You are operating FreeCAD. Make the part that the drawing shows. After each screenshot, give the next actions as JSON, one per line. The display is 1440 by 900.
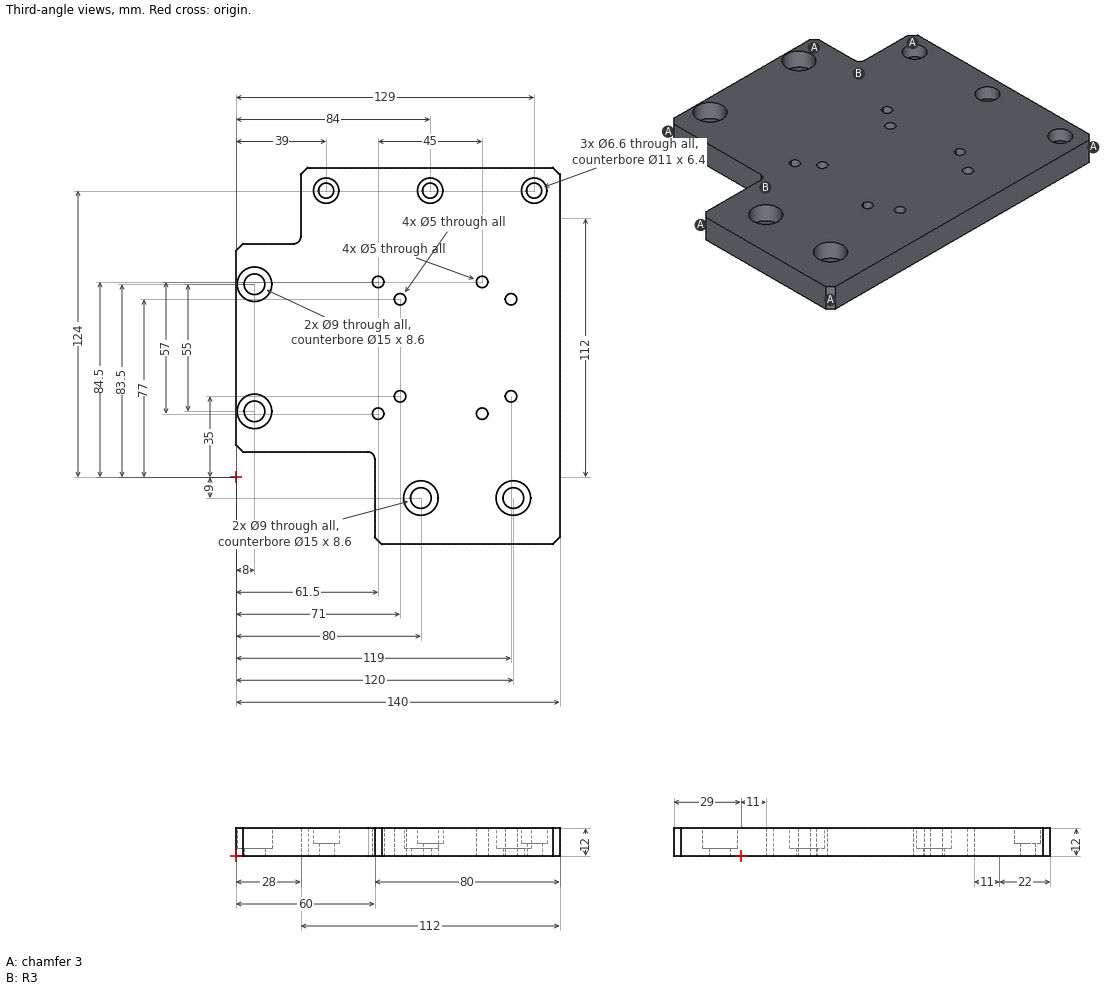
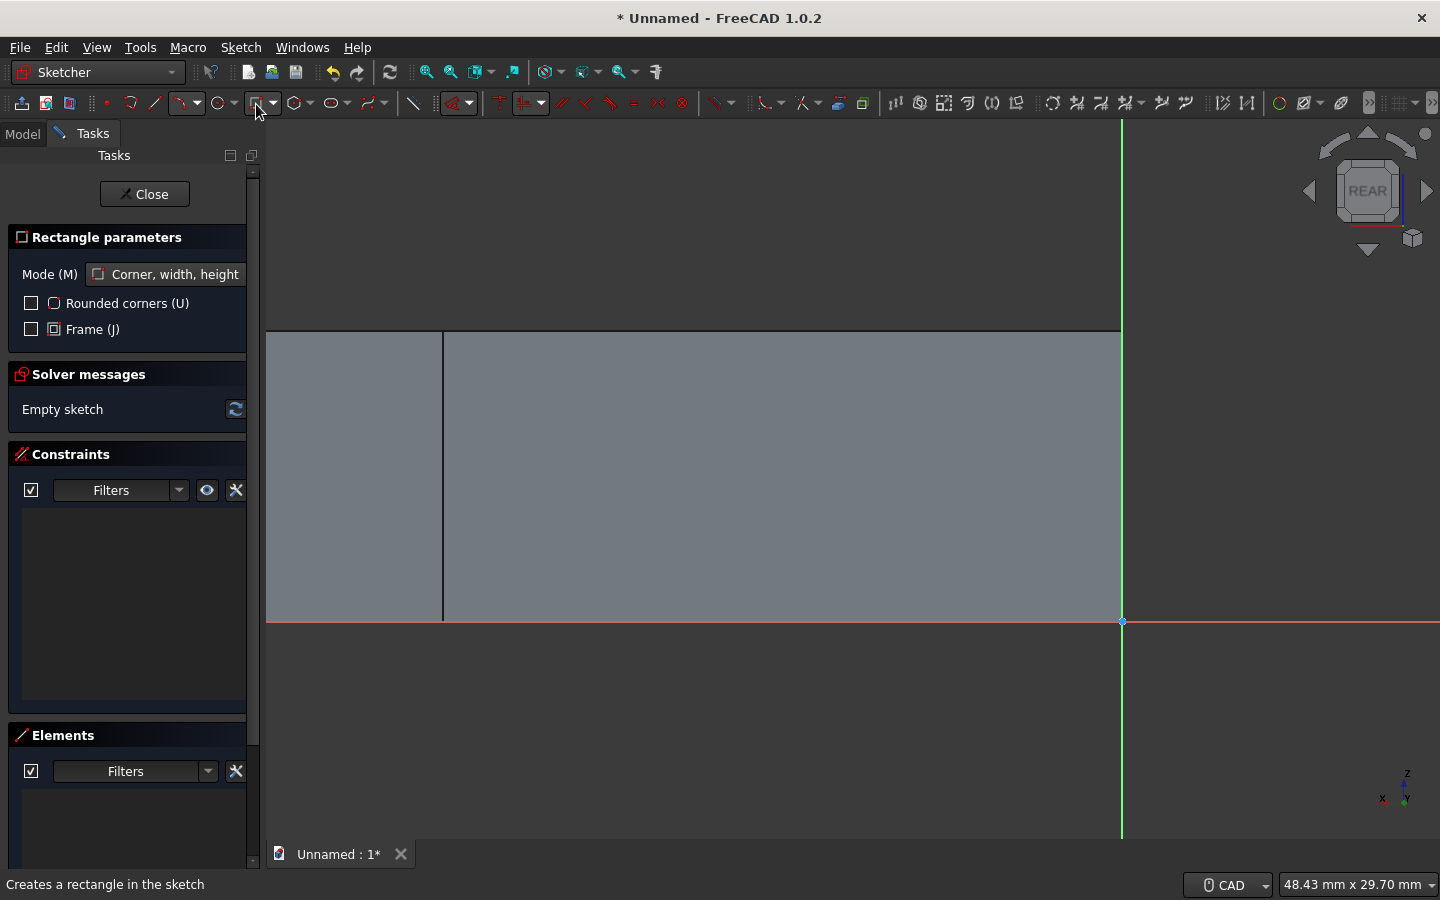
{"action": "left_click", "coordinate": [1122, 622]}
{"action": "mouse_move", "coordinate": [443, 331]}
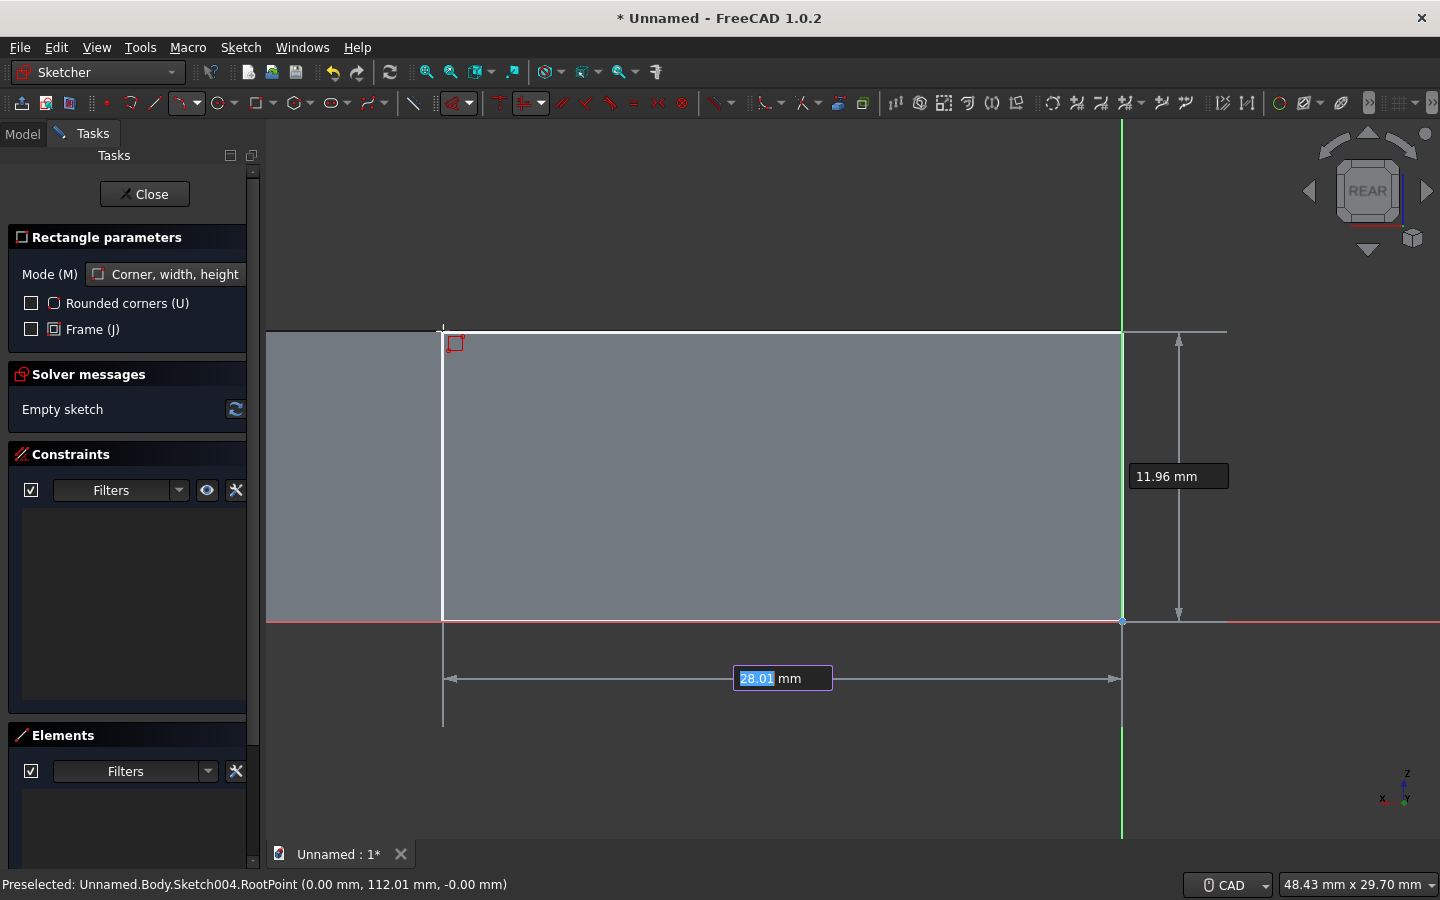
{"action": "type", "text": "28"}
{"action": "key", "text": "Tab"}
{"action": "type", "text": "12"}
{"action": "key", "text": "Return"}
{"action": "key", "text": "Escape"}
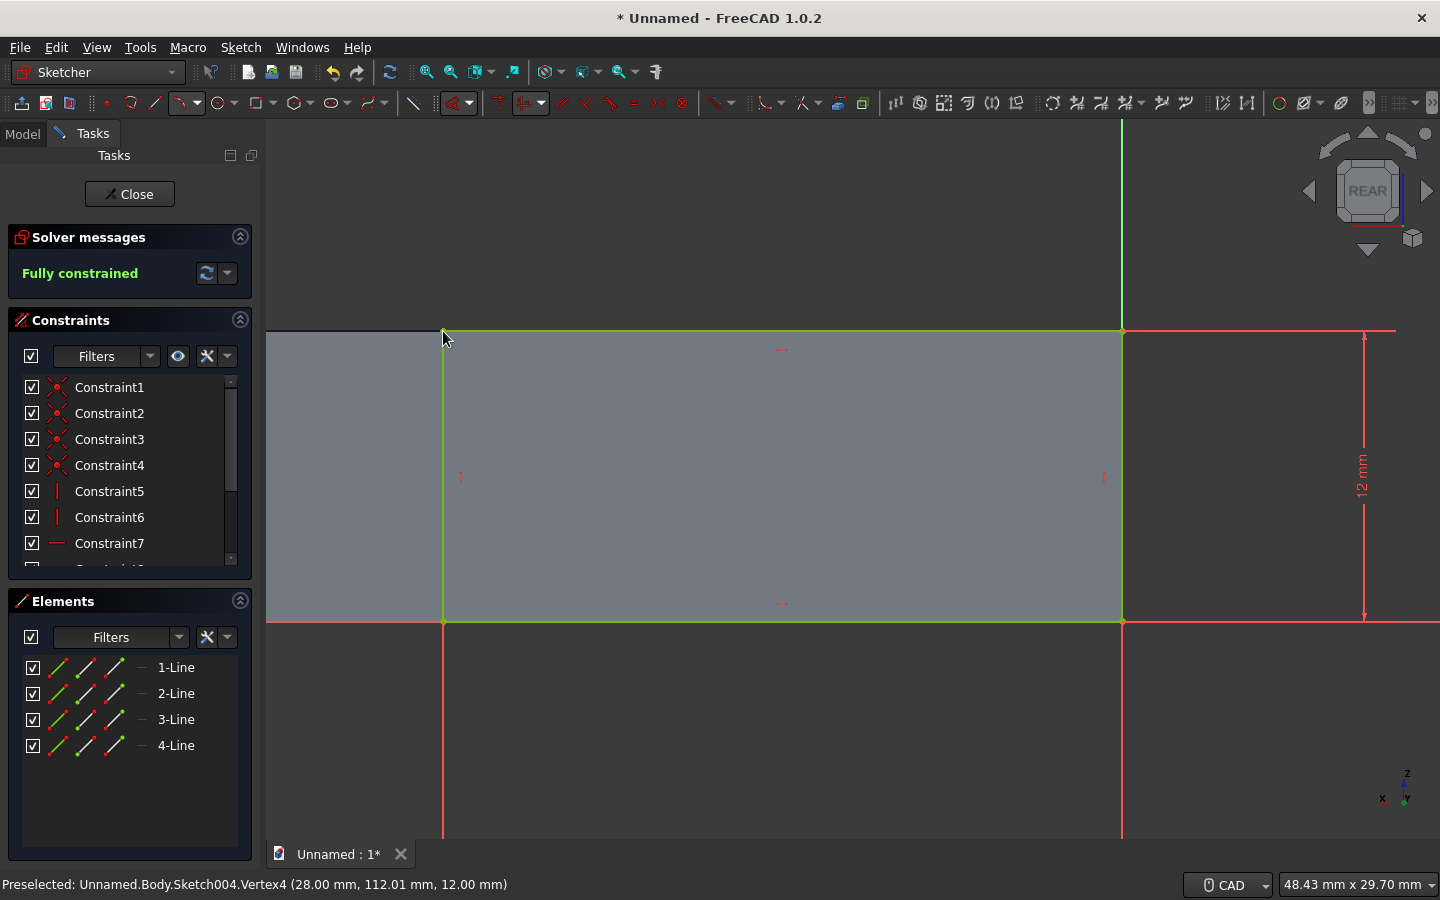
{"action": "left_click", "coordinate": [130, 194]}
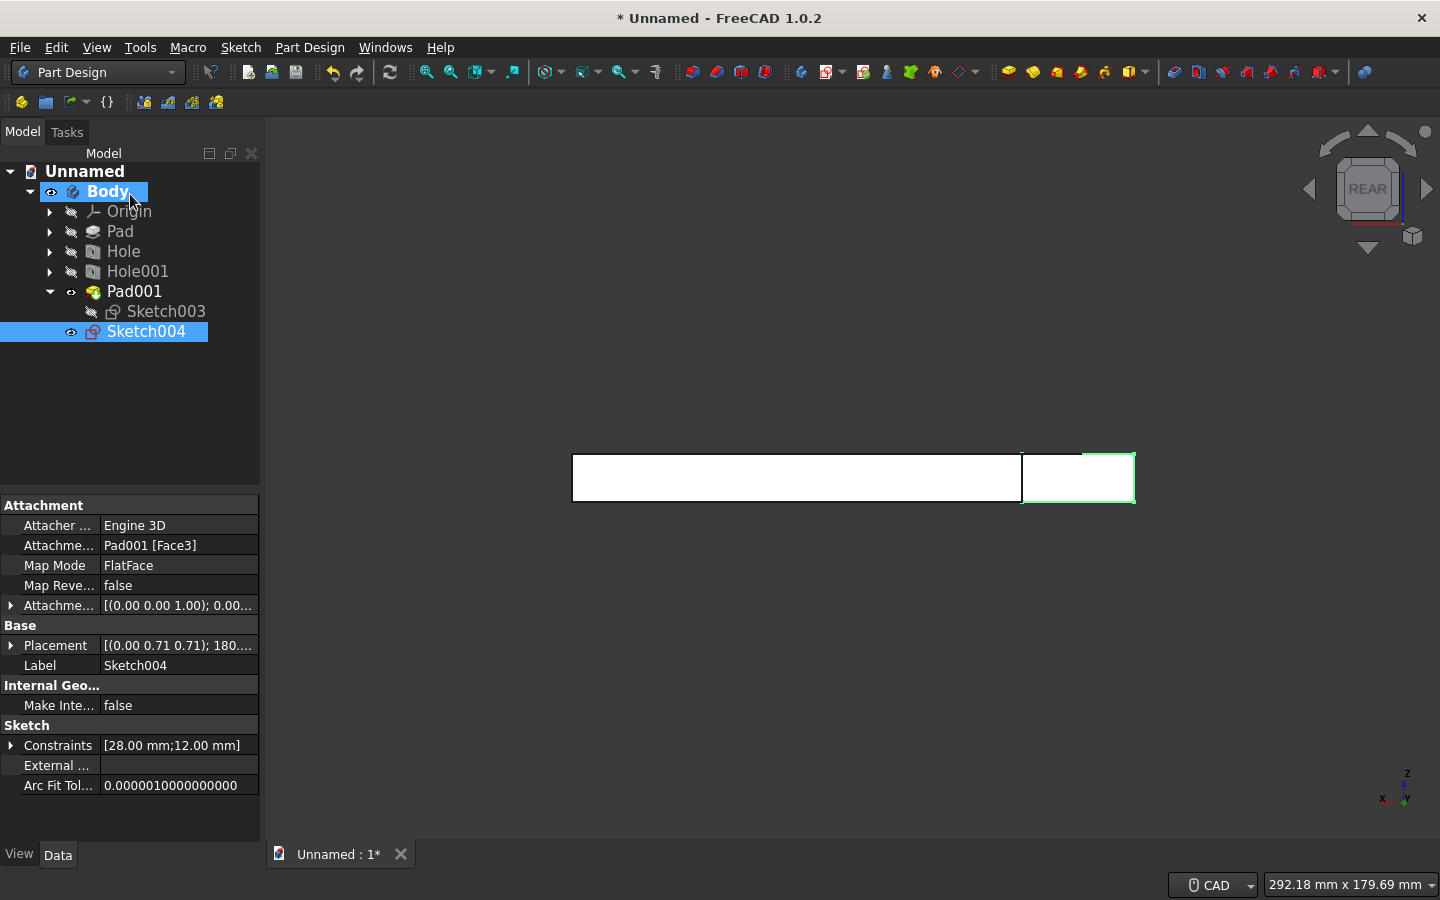
{"action": "left_click", "coordinate": [1176, 72]}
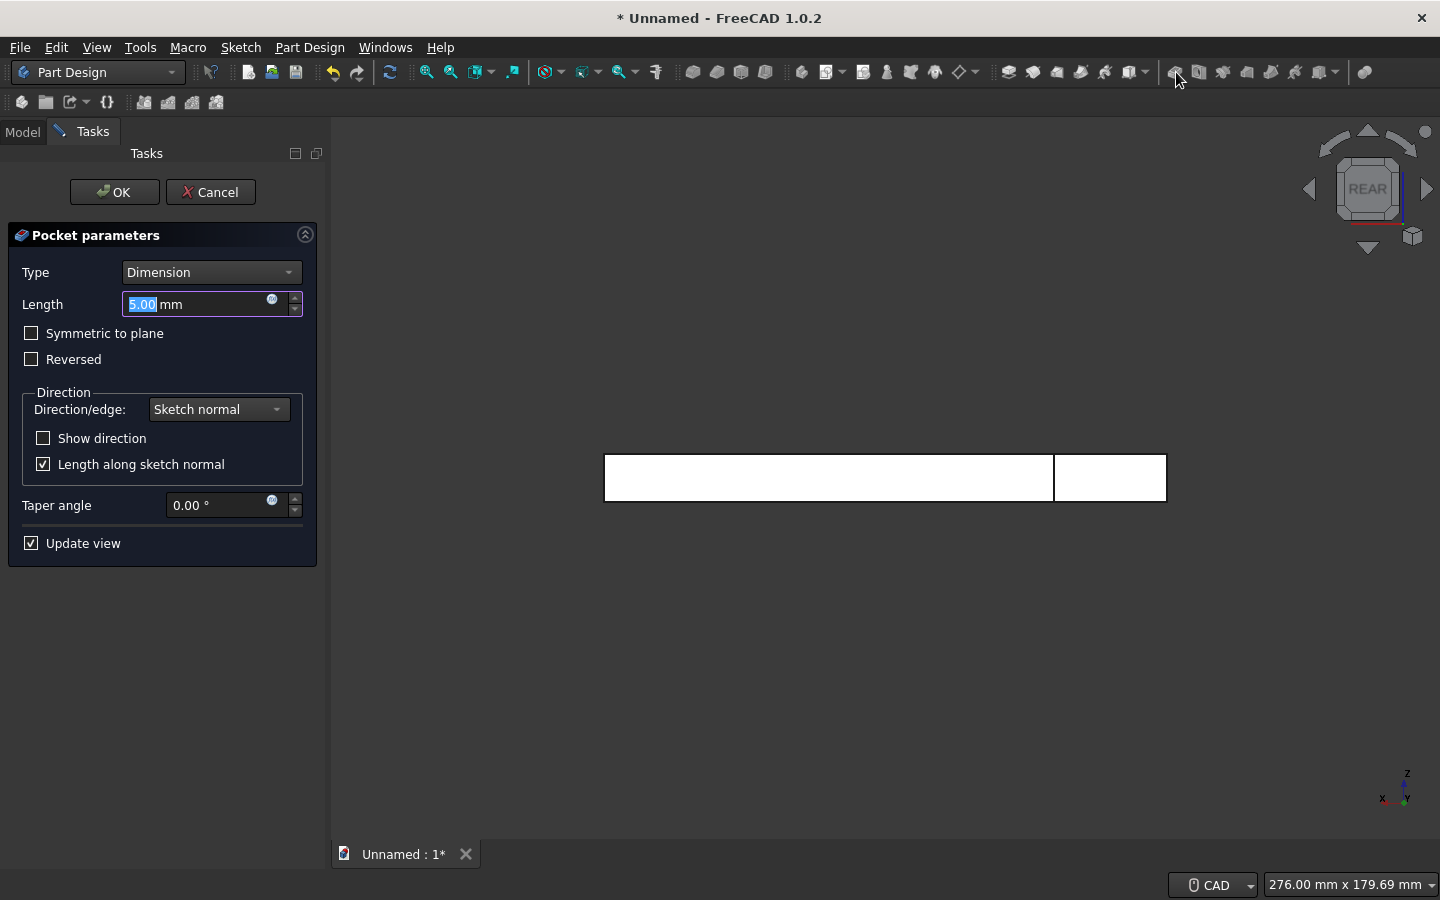
{"action": "type", "text": "11"}
{"action": "key", "text": "Tab"}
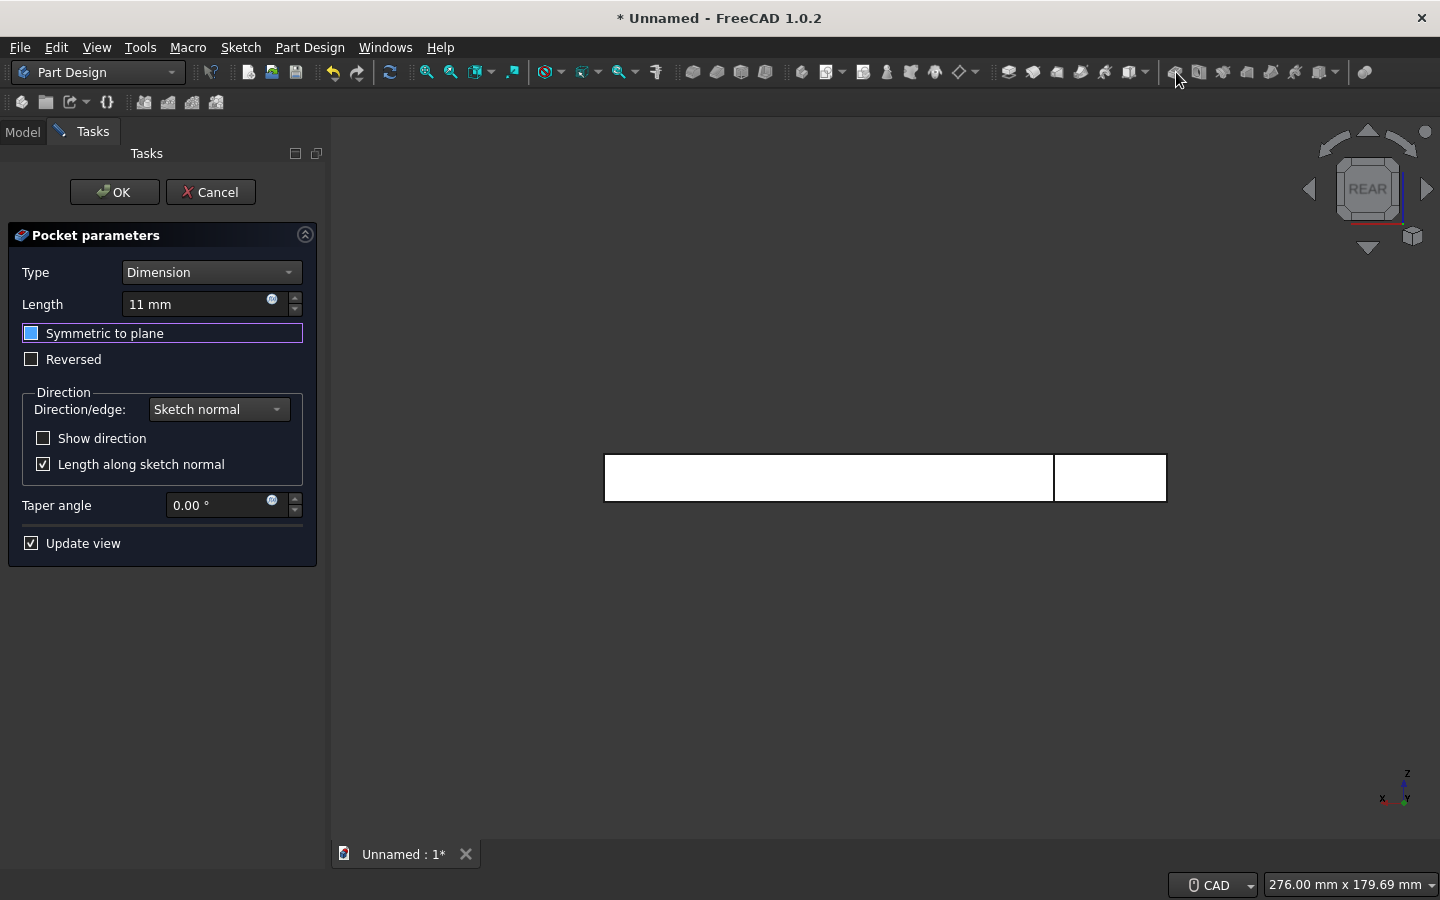
{"action": "left_click", "coordinate": [115, 192]}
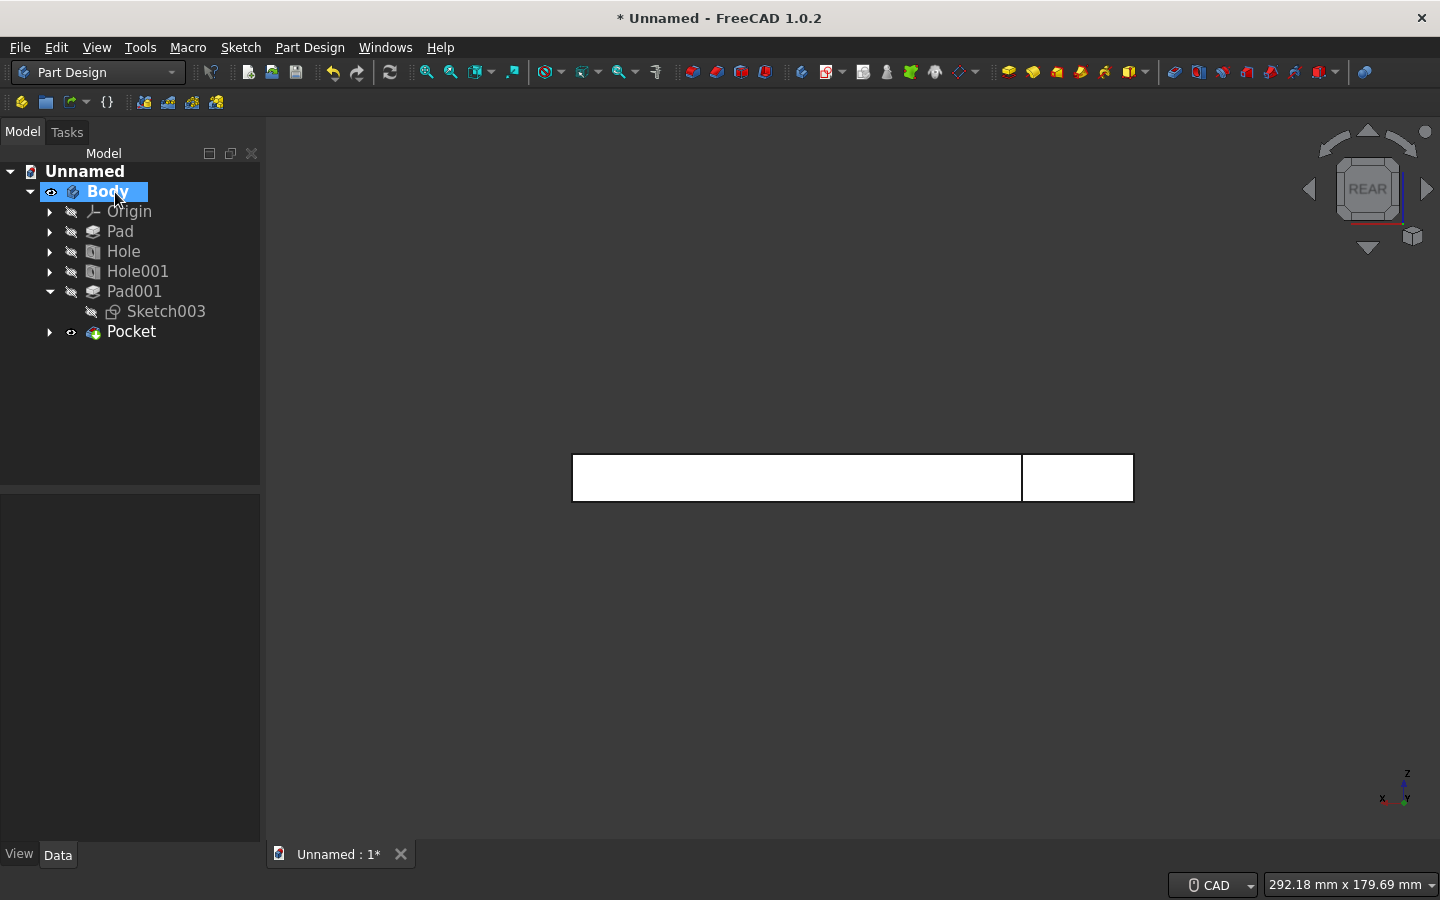
{"action": "key", "text": "0"}